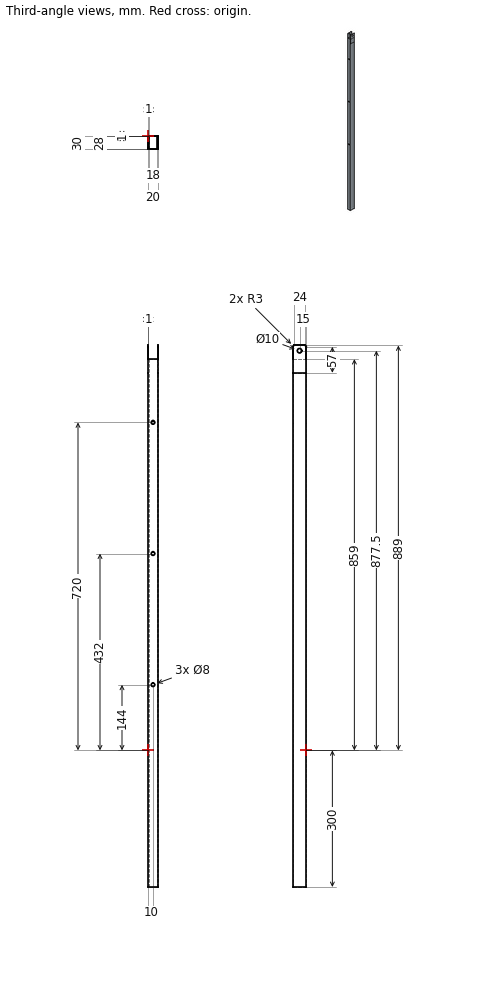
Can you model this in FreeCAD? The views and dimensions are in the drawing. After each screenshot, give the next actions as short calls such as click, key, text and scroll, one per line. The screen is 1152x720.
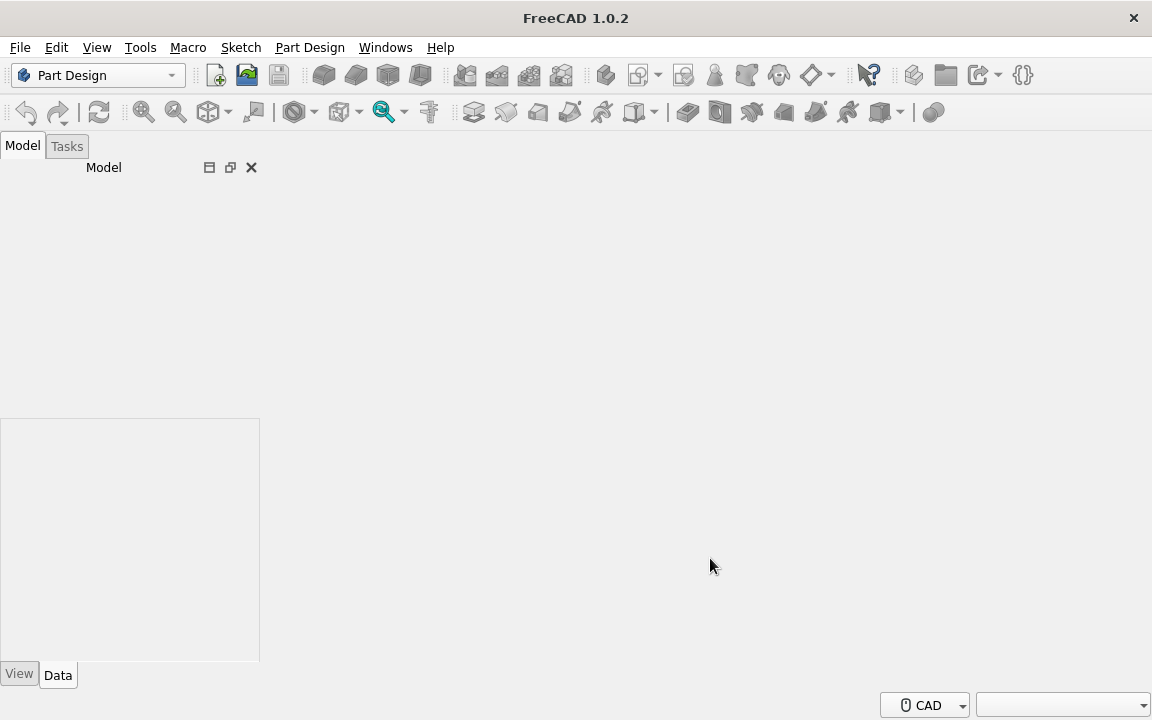
key(ctrl+n)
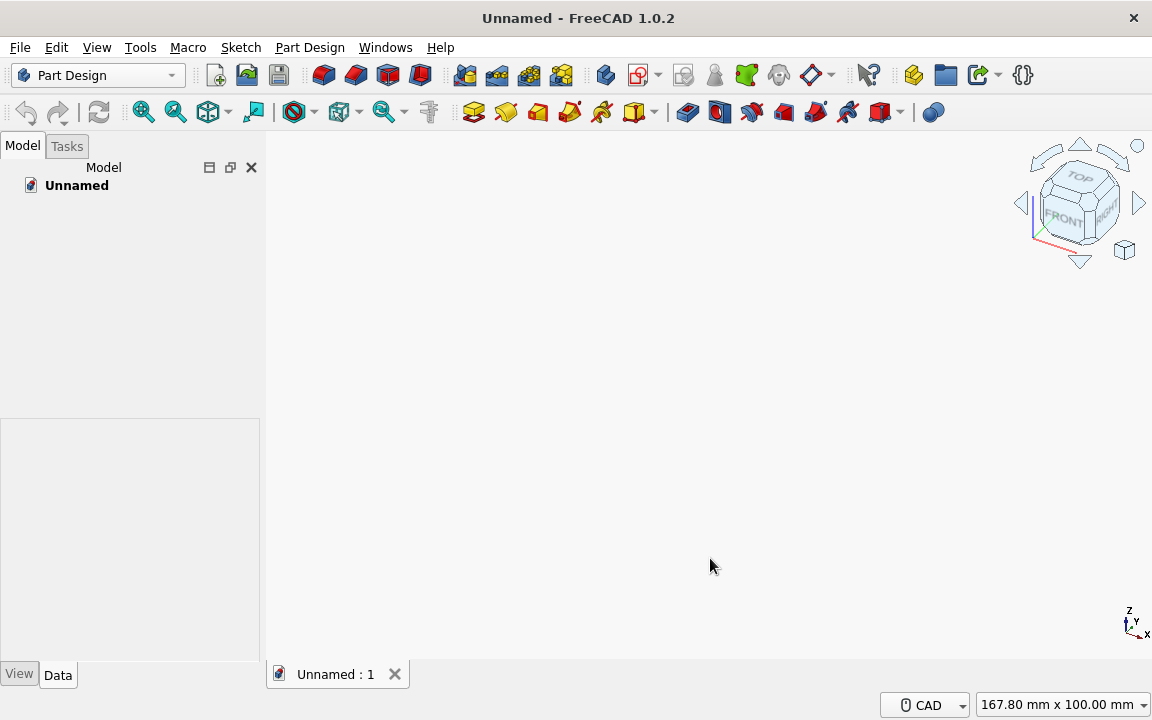
click(638, 76)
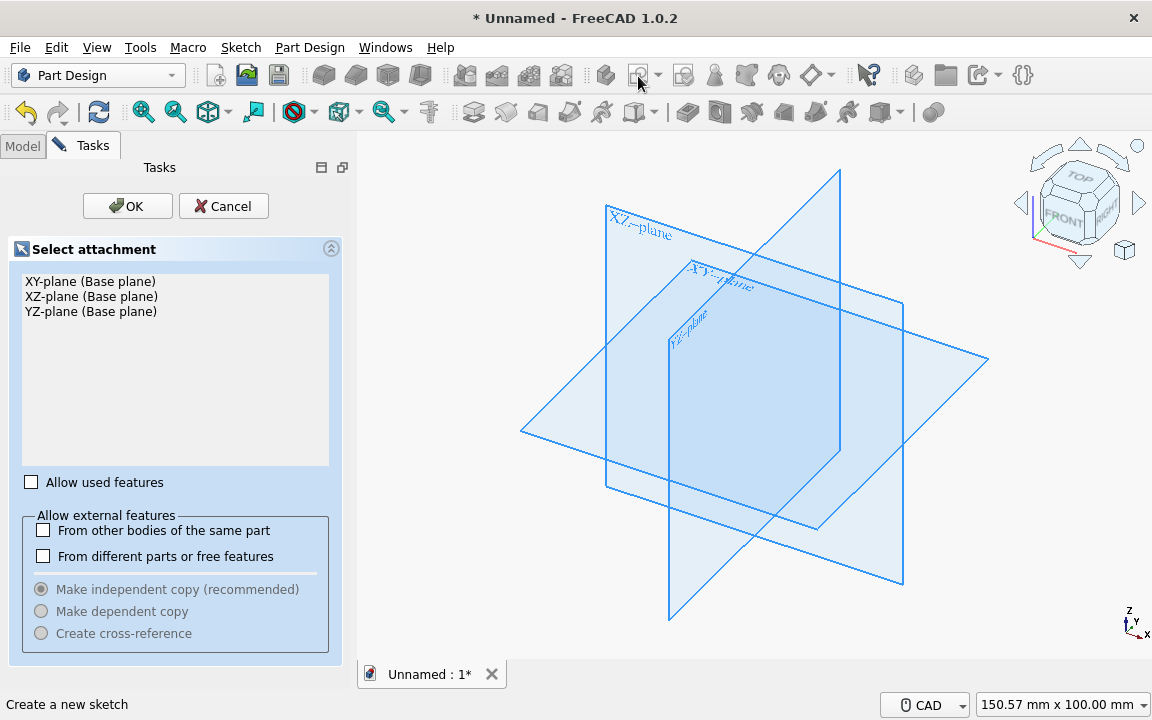
click(82, 282)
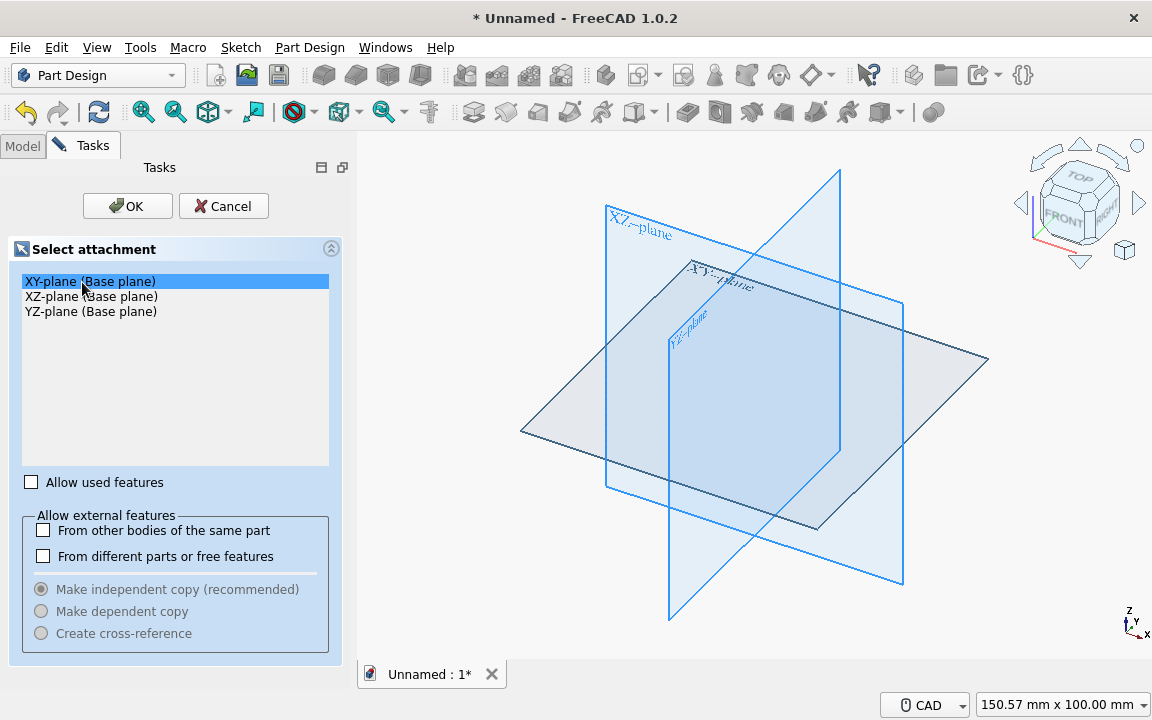
click(128, 206)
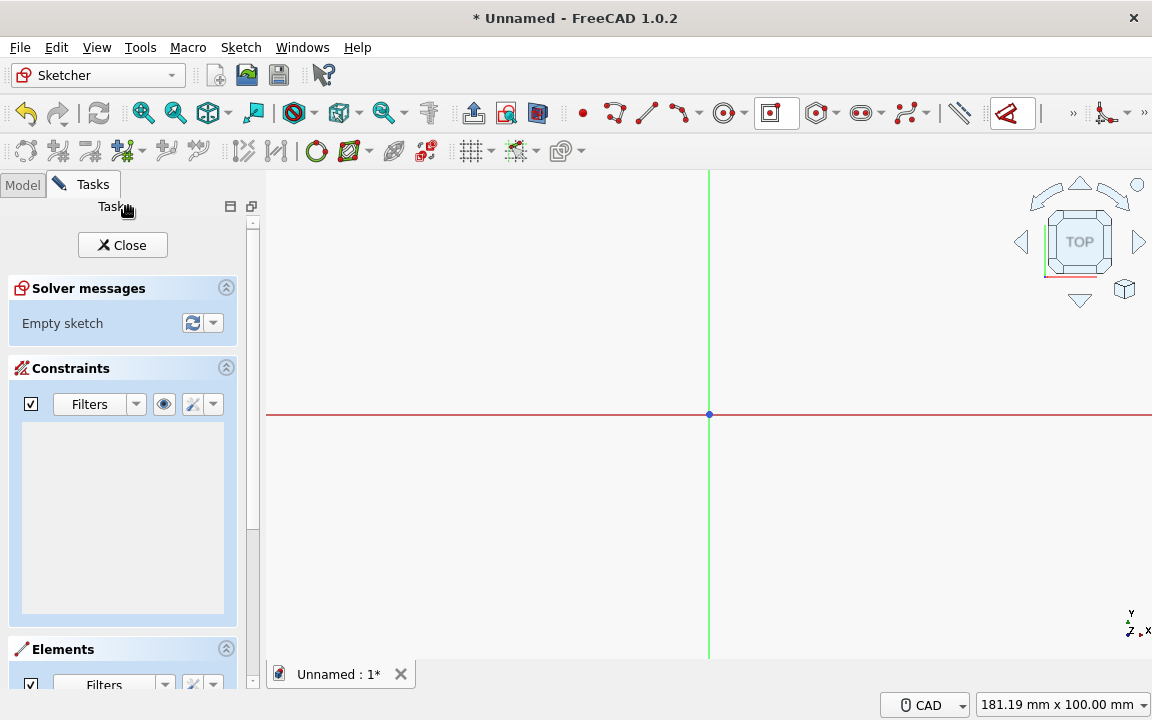
scroll(854, 548, up, 4)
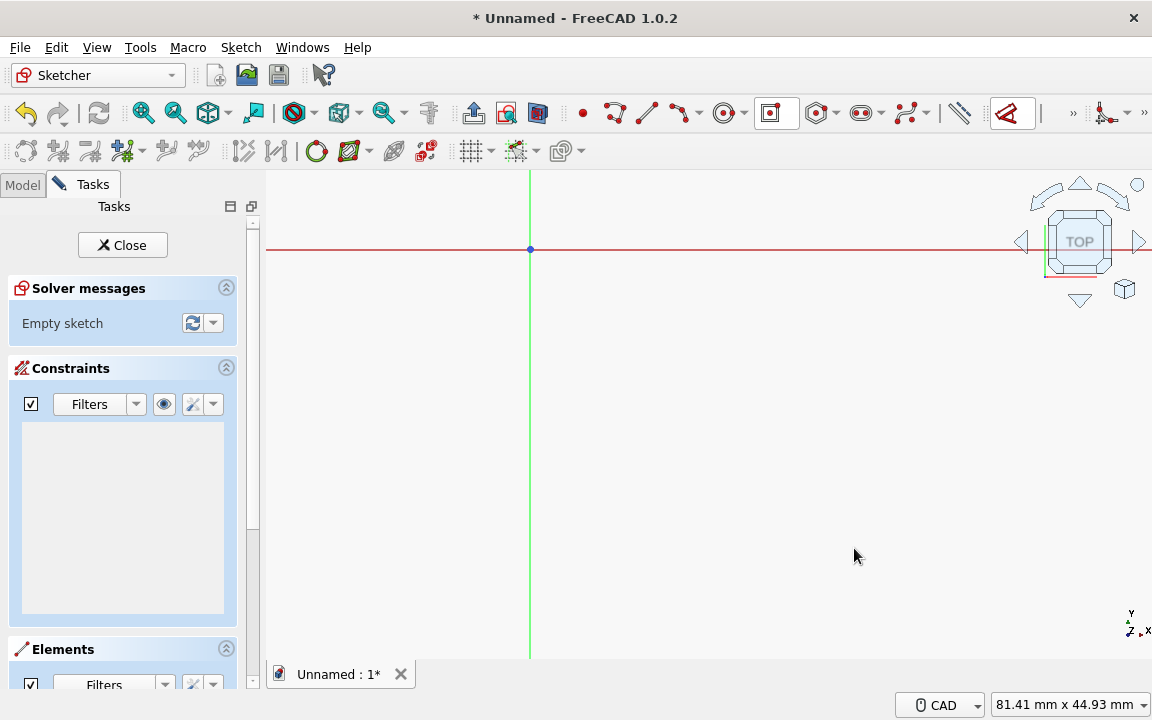
key(g)
key(r)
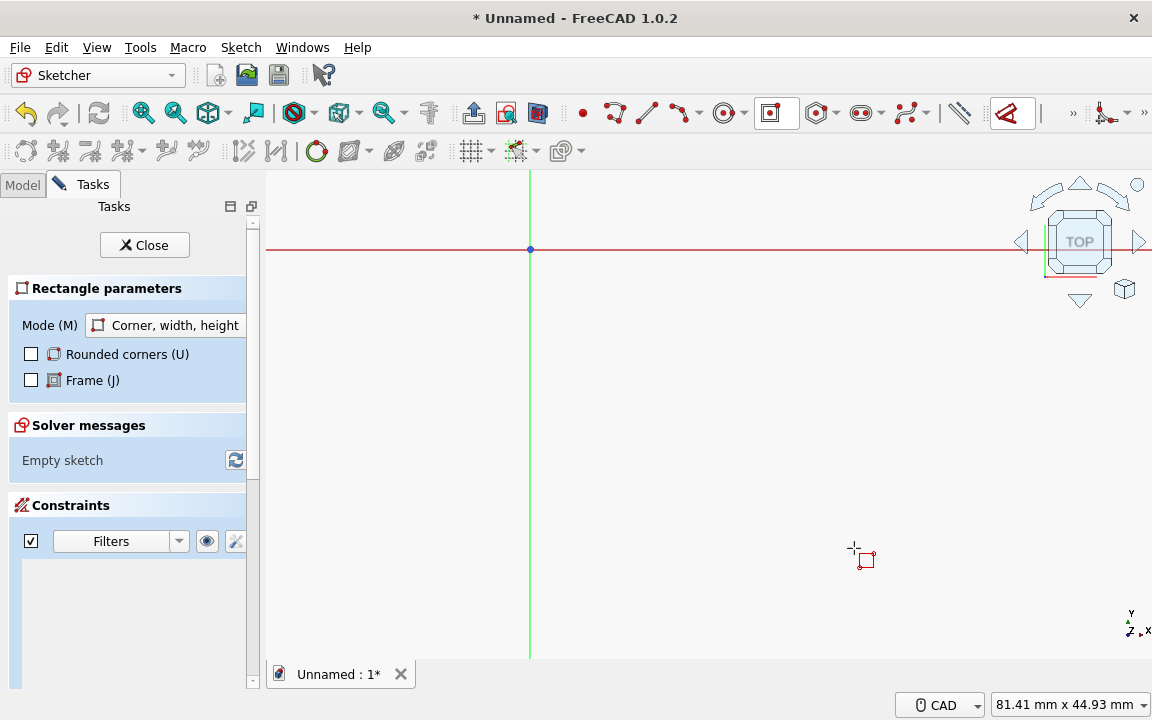
click(530, 250)
click(748, 576)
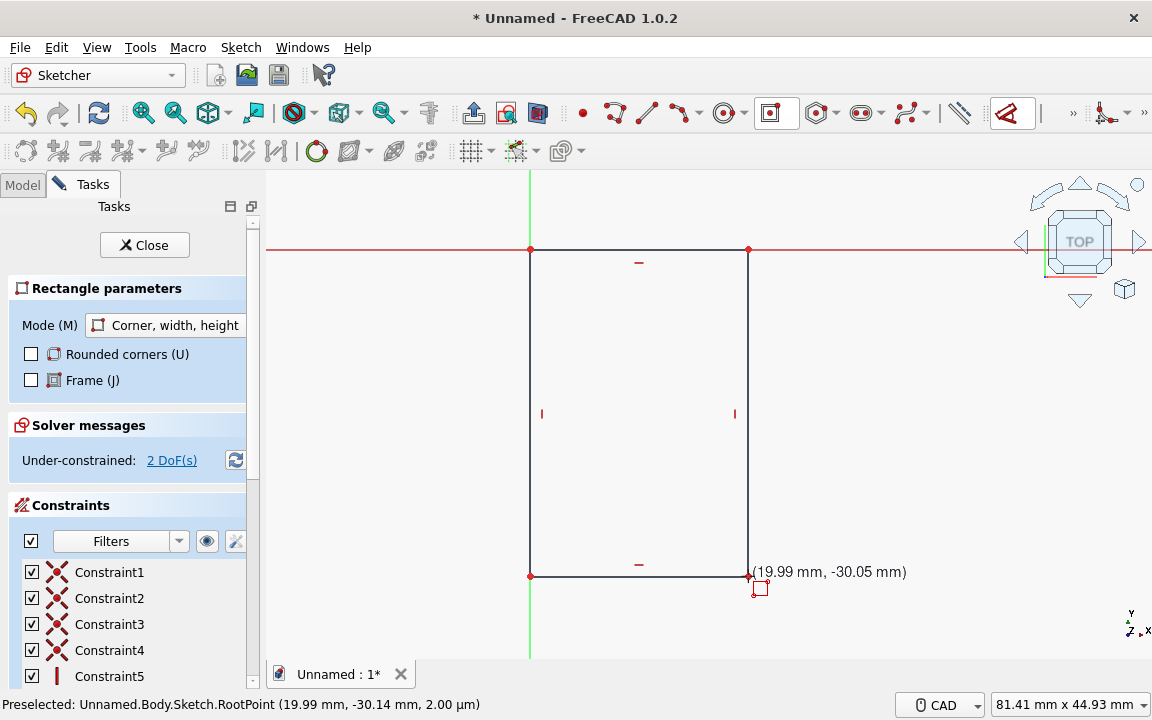
scroll(541, 261, up, 2)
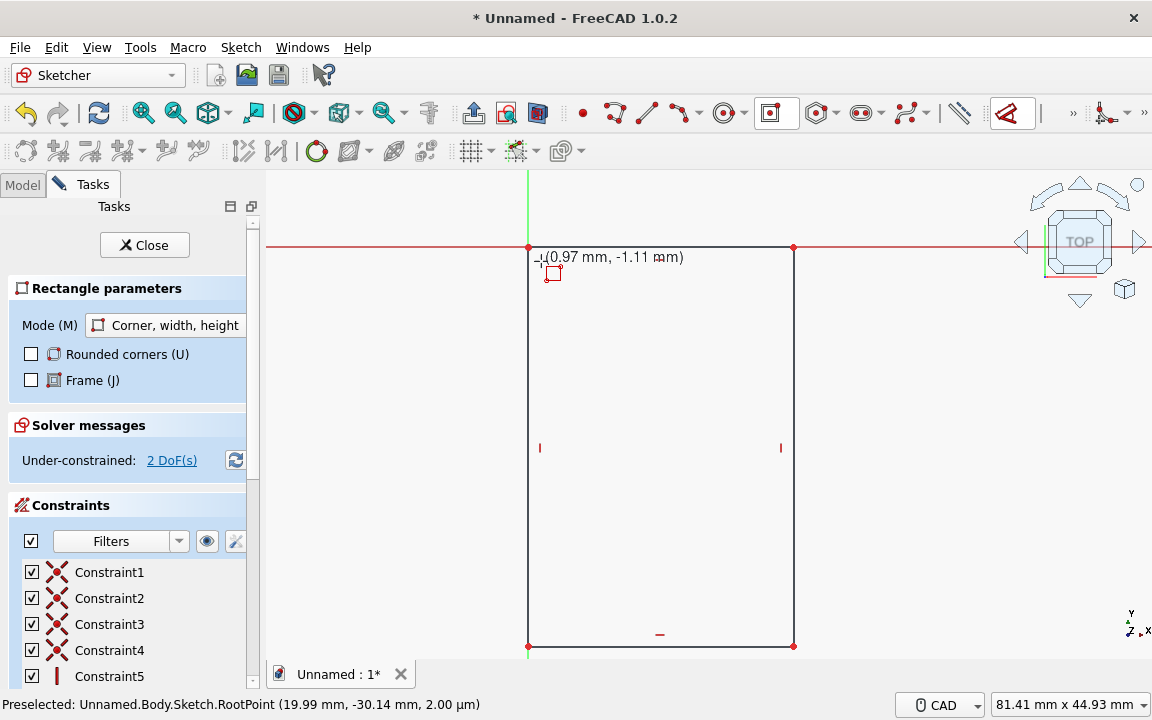
click(541, 261)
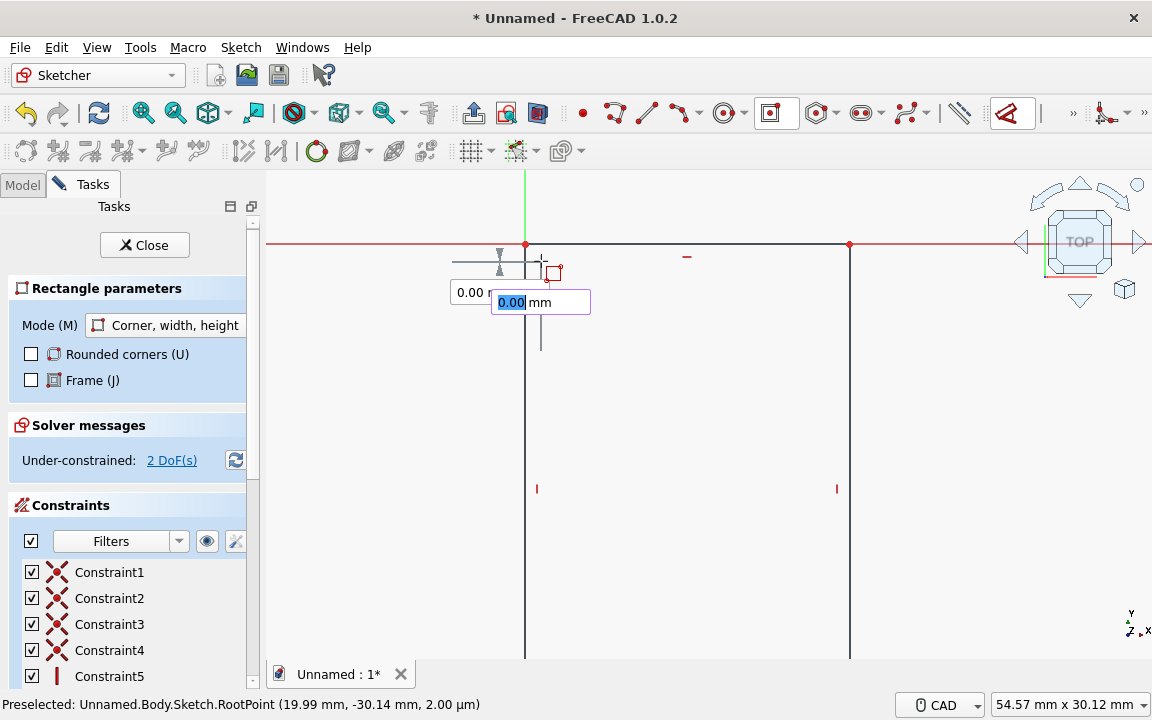
scroll(545, 265, down, 2)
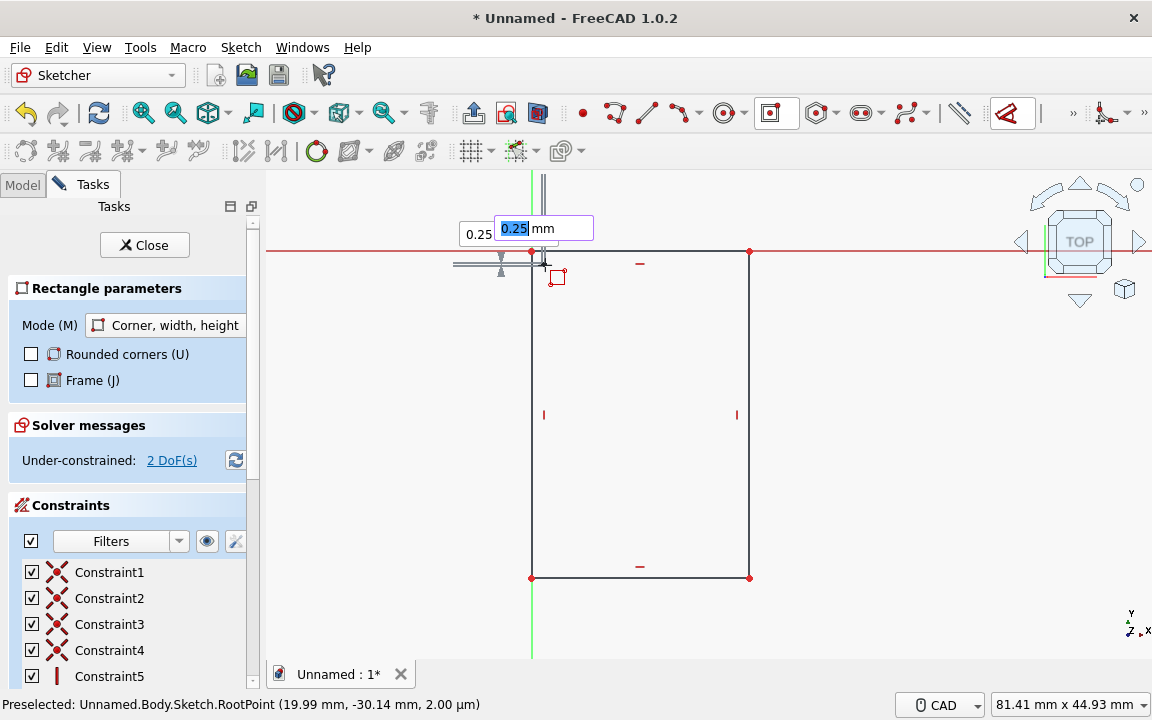
scroll(739, 567, up, 2)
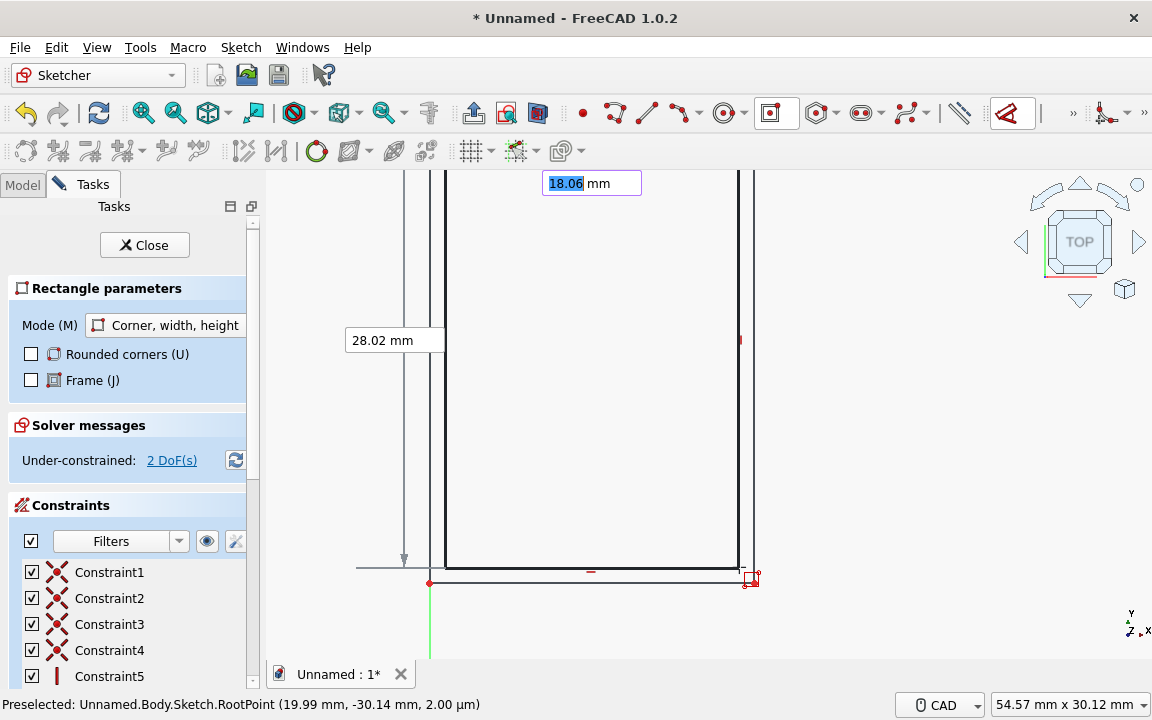
click(738, 566)
key(Escape)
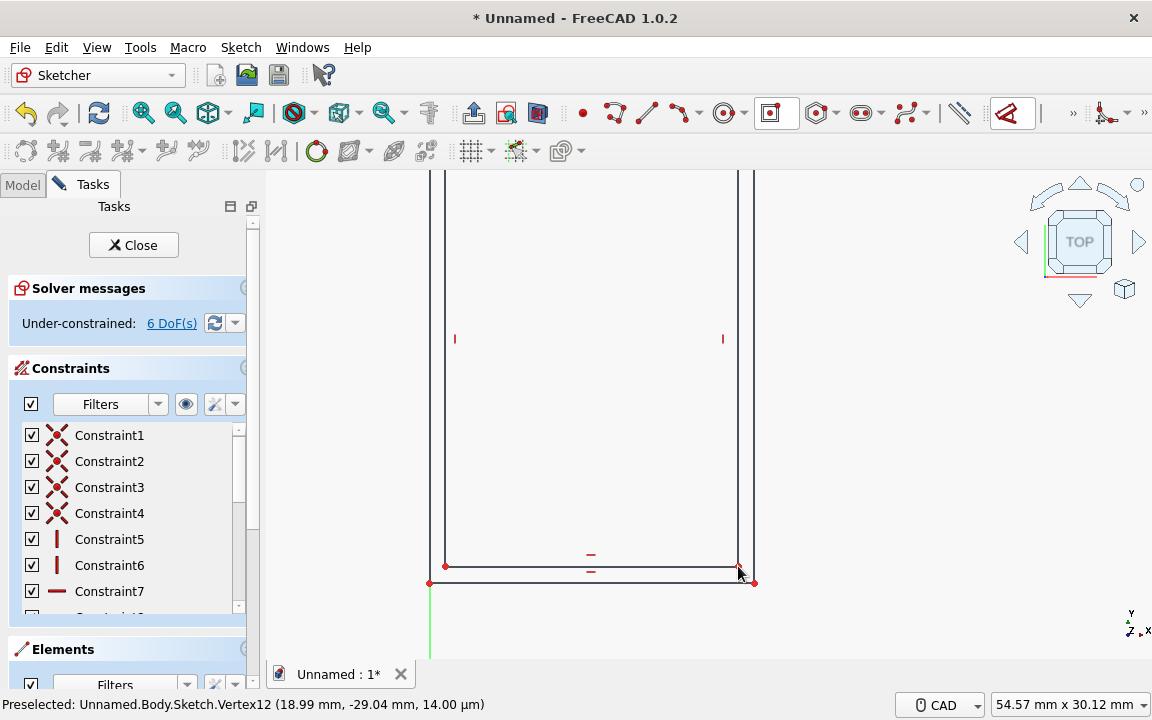
click(430, 242)